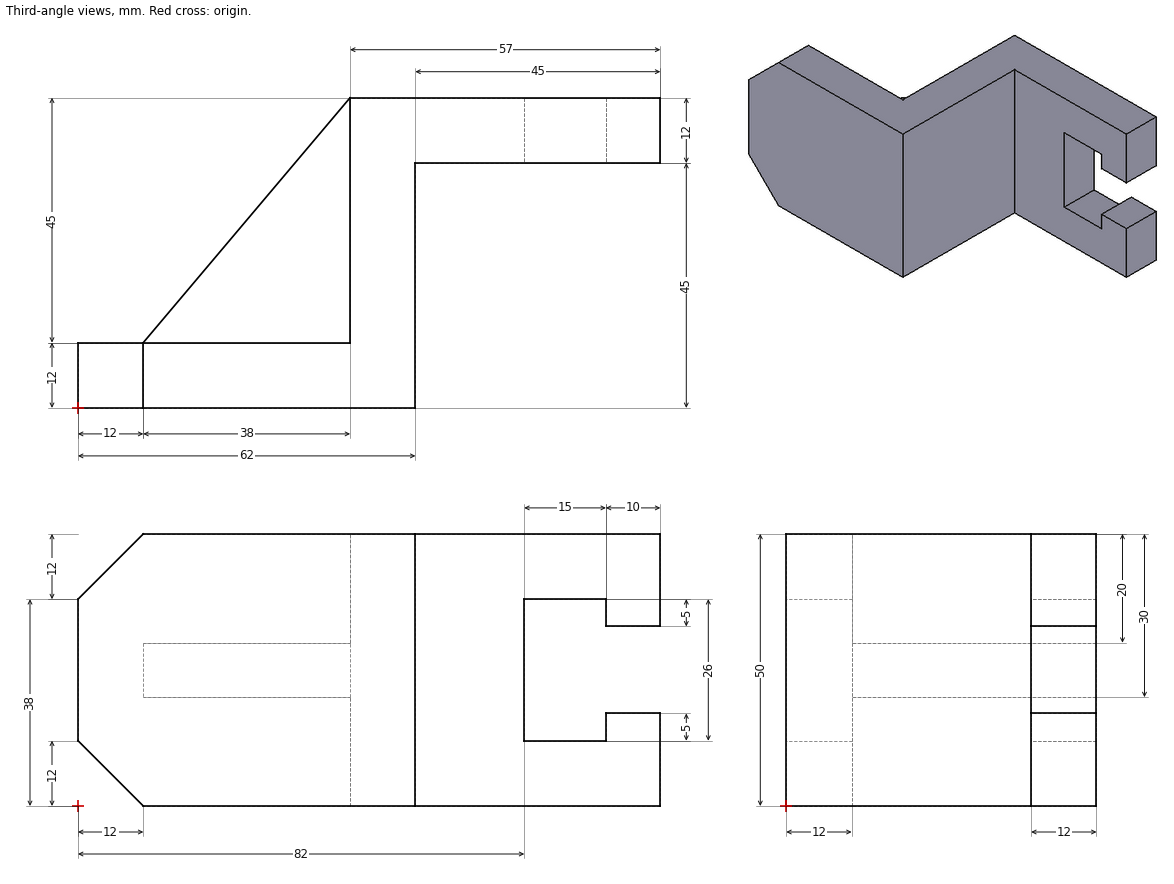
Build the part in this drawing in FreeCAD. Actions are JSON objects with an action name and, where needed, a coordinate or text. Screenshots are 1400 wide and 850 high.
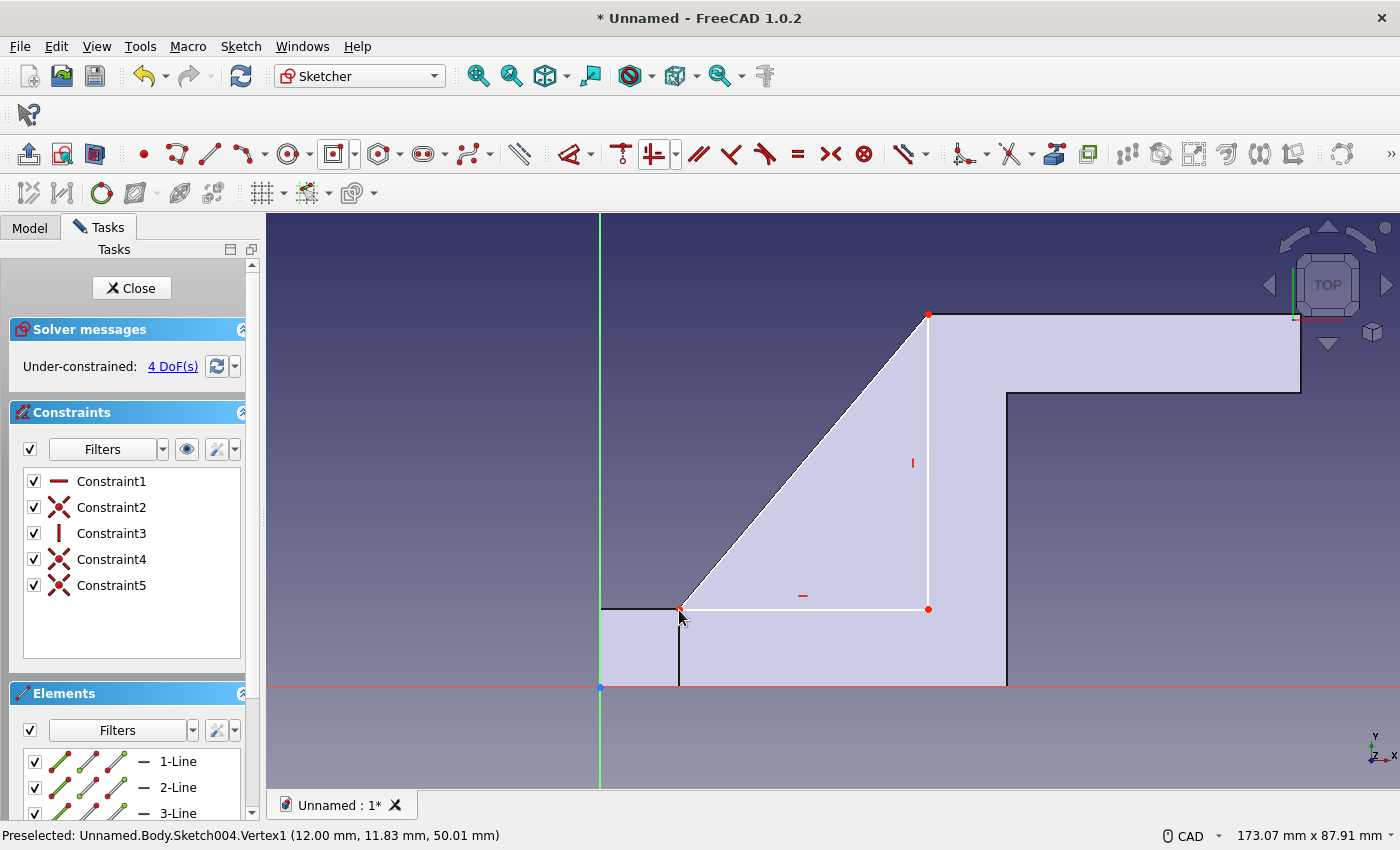
{"action": "left_click", "coordinate": [568, 154]}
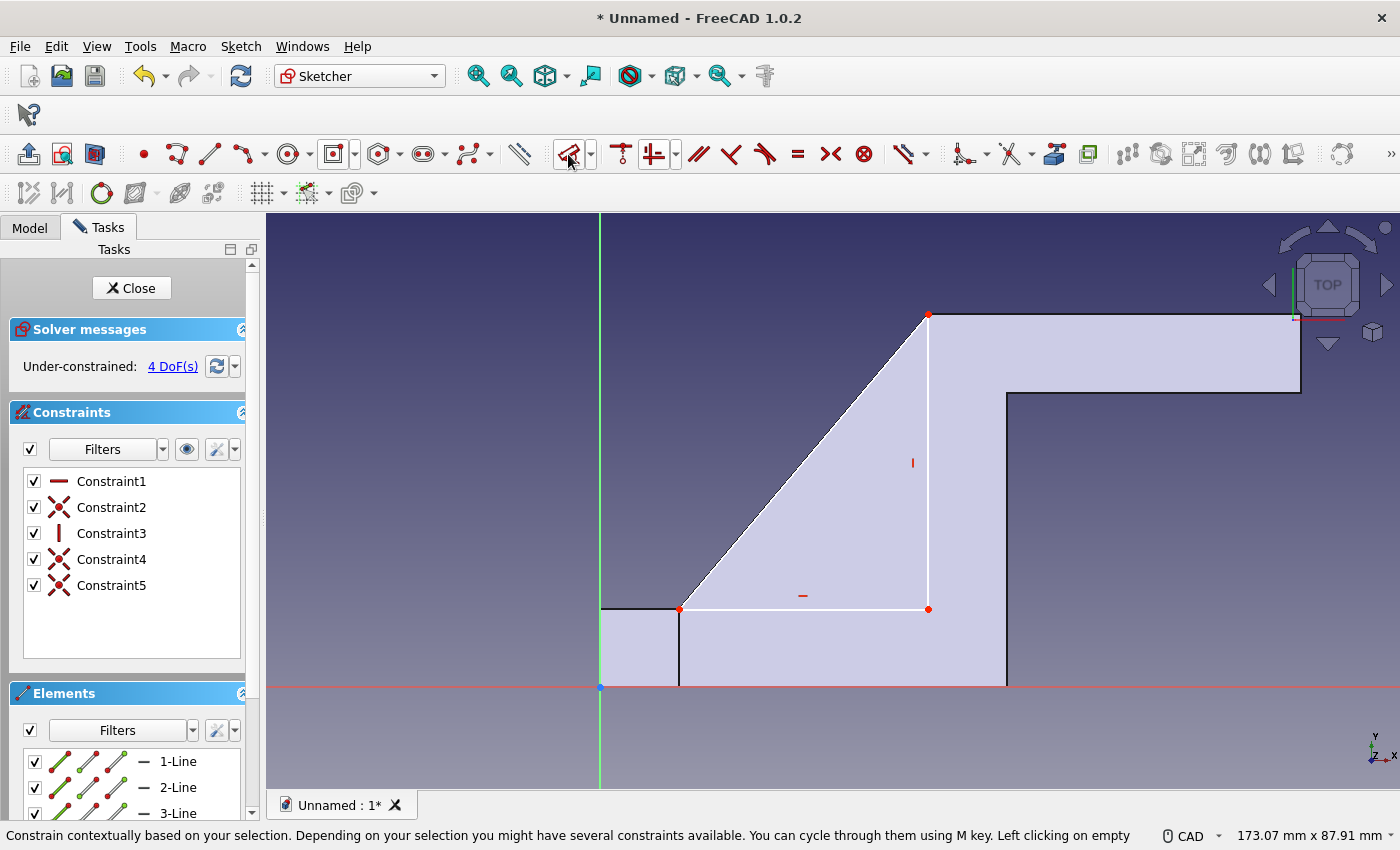
{"action": "left_click", "coordinate": [754, 610]}
{"action": "left_click", "coordinate": [803, 644]}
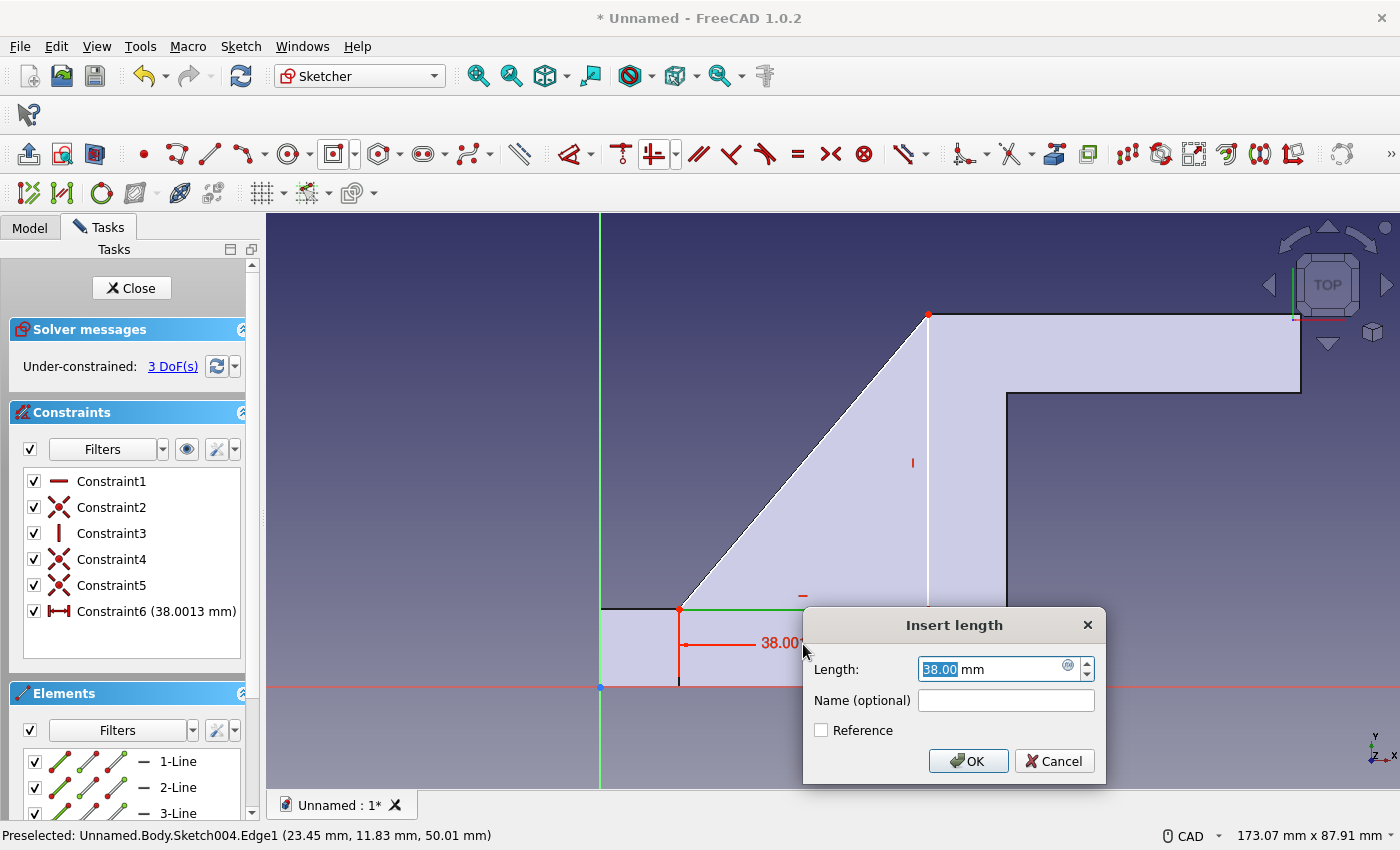
{"action": "type", "text": "38"}
{"action": "key", "text": "Return"}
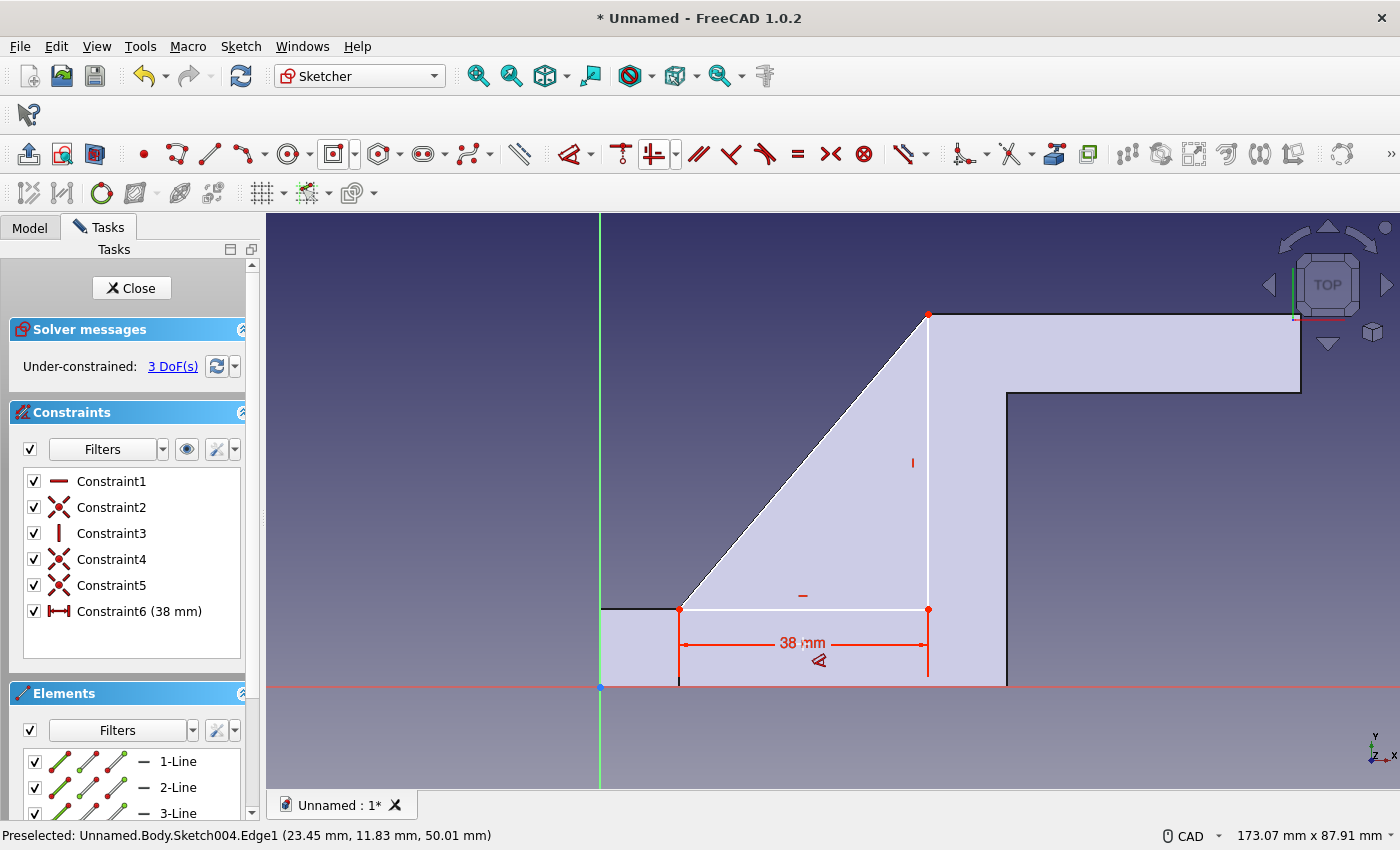
{"action": "left_click", "coordinate": [928, 521]}
{"action": "left_click", "coordinate": [962, 462]}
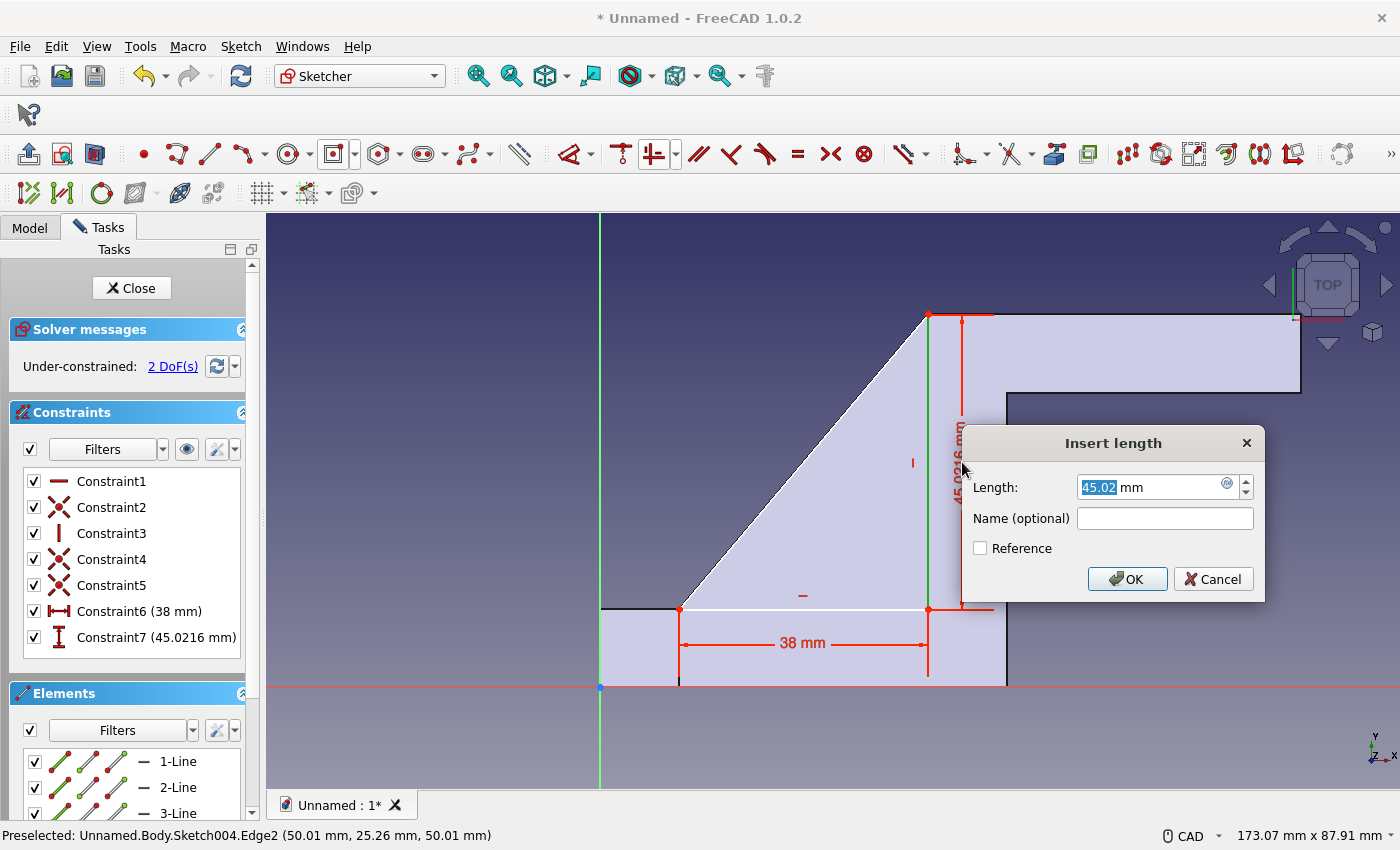
{"action": "type", "text": "45"}
{"action": "key", "text": "Return"}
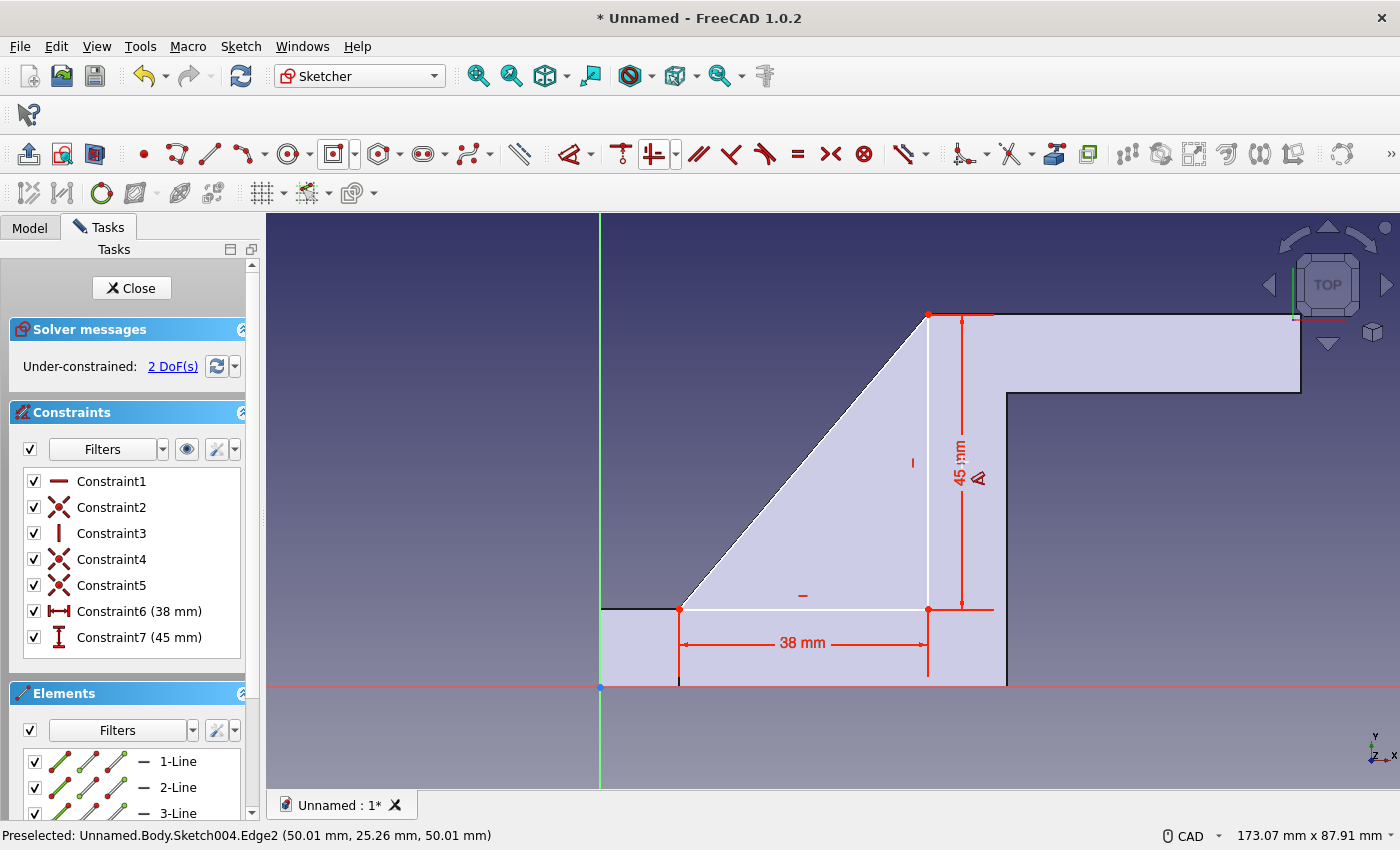
{"action": "left_click", "coordinate": [679, 610]}
{"action": "left_click", "coordinate": [640, 721]}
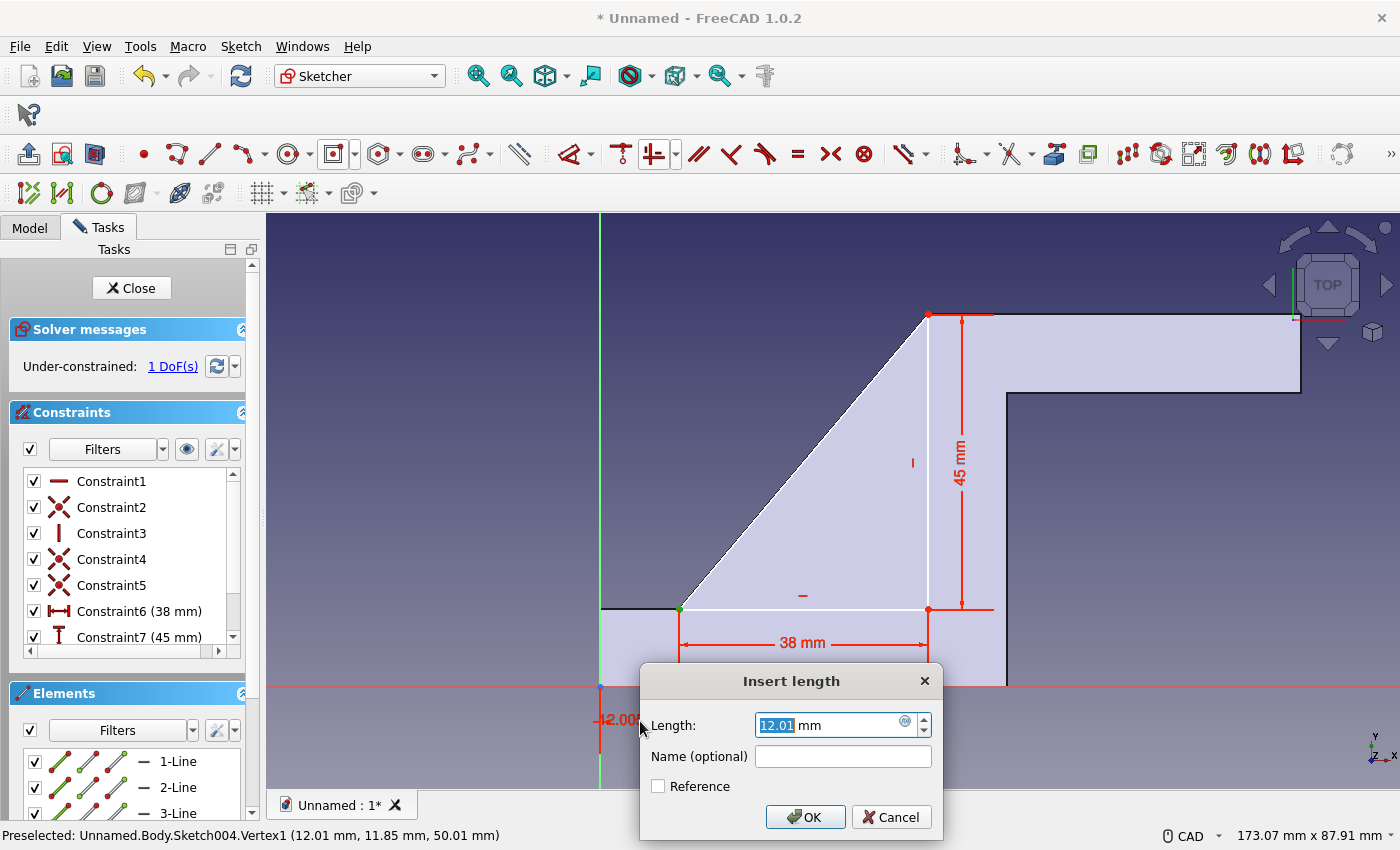
{"action": "type", "text": "12"}
{"action": "key", "text": "Return"}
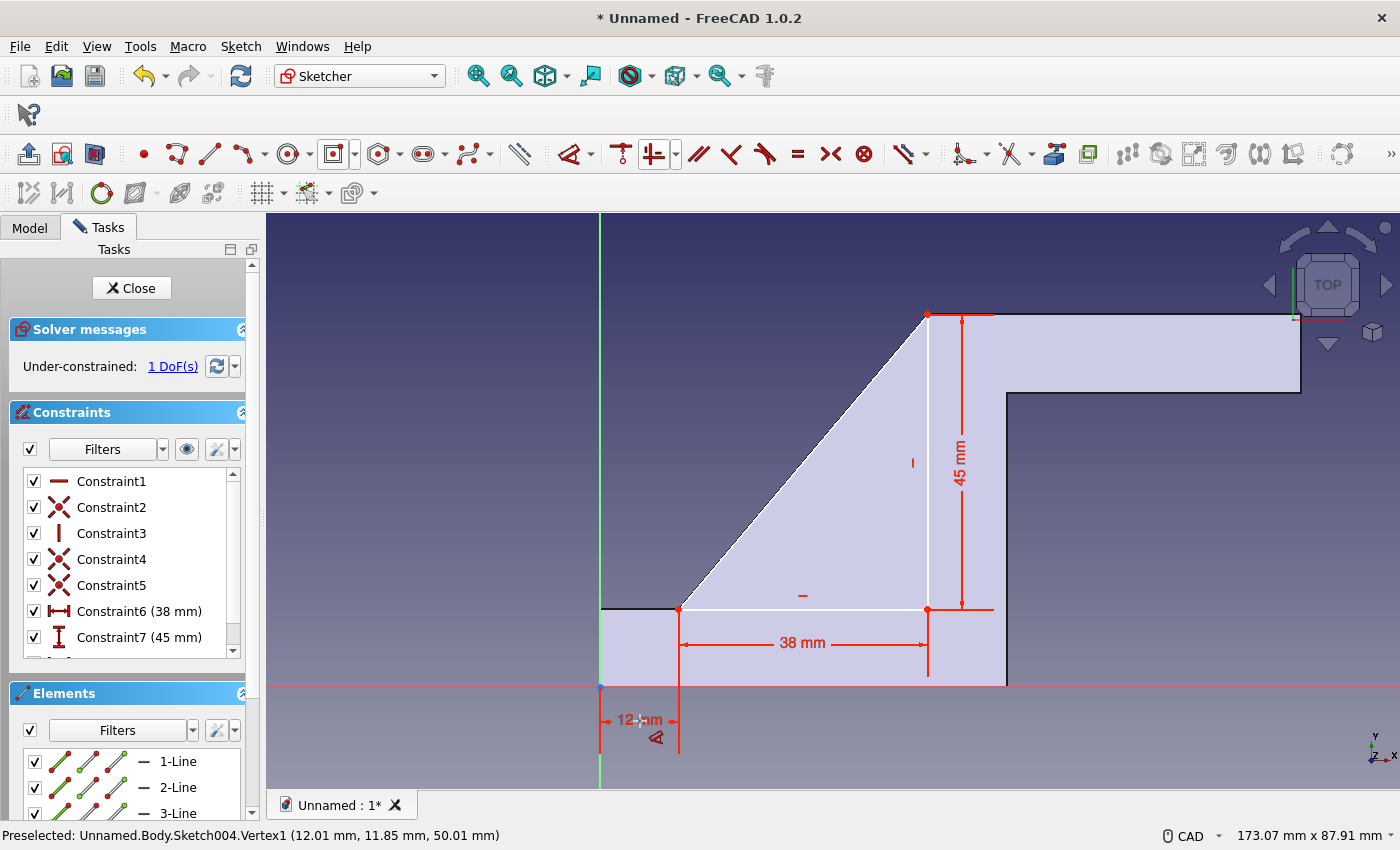
{"action": "left_click", "coordinate": [679, 610]}
{"action": "left_click", "coordinate": [566, 649]}